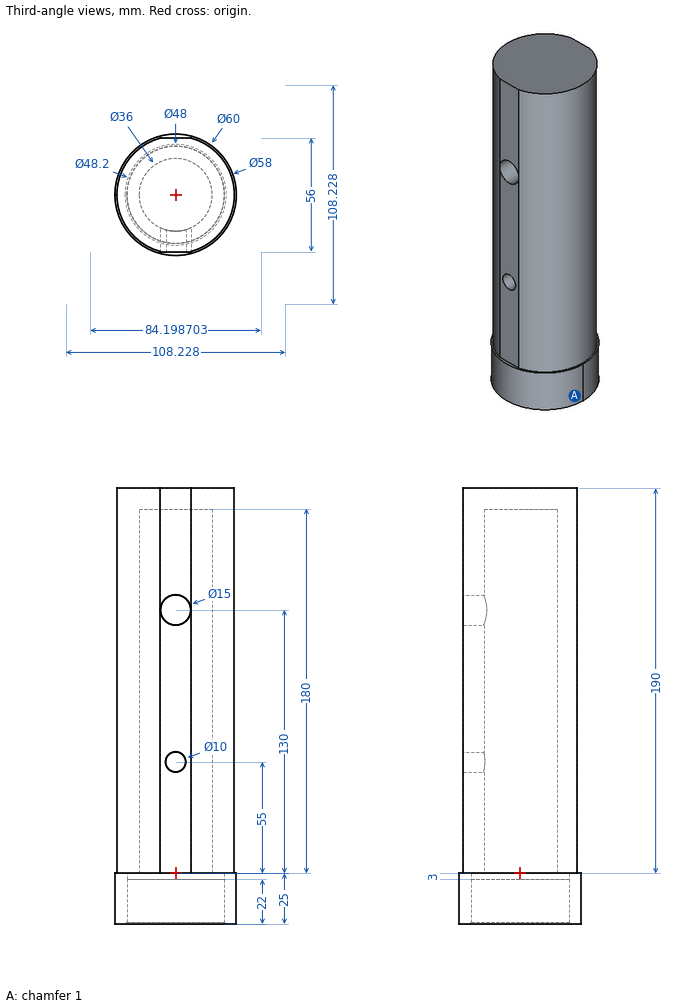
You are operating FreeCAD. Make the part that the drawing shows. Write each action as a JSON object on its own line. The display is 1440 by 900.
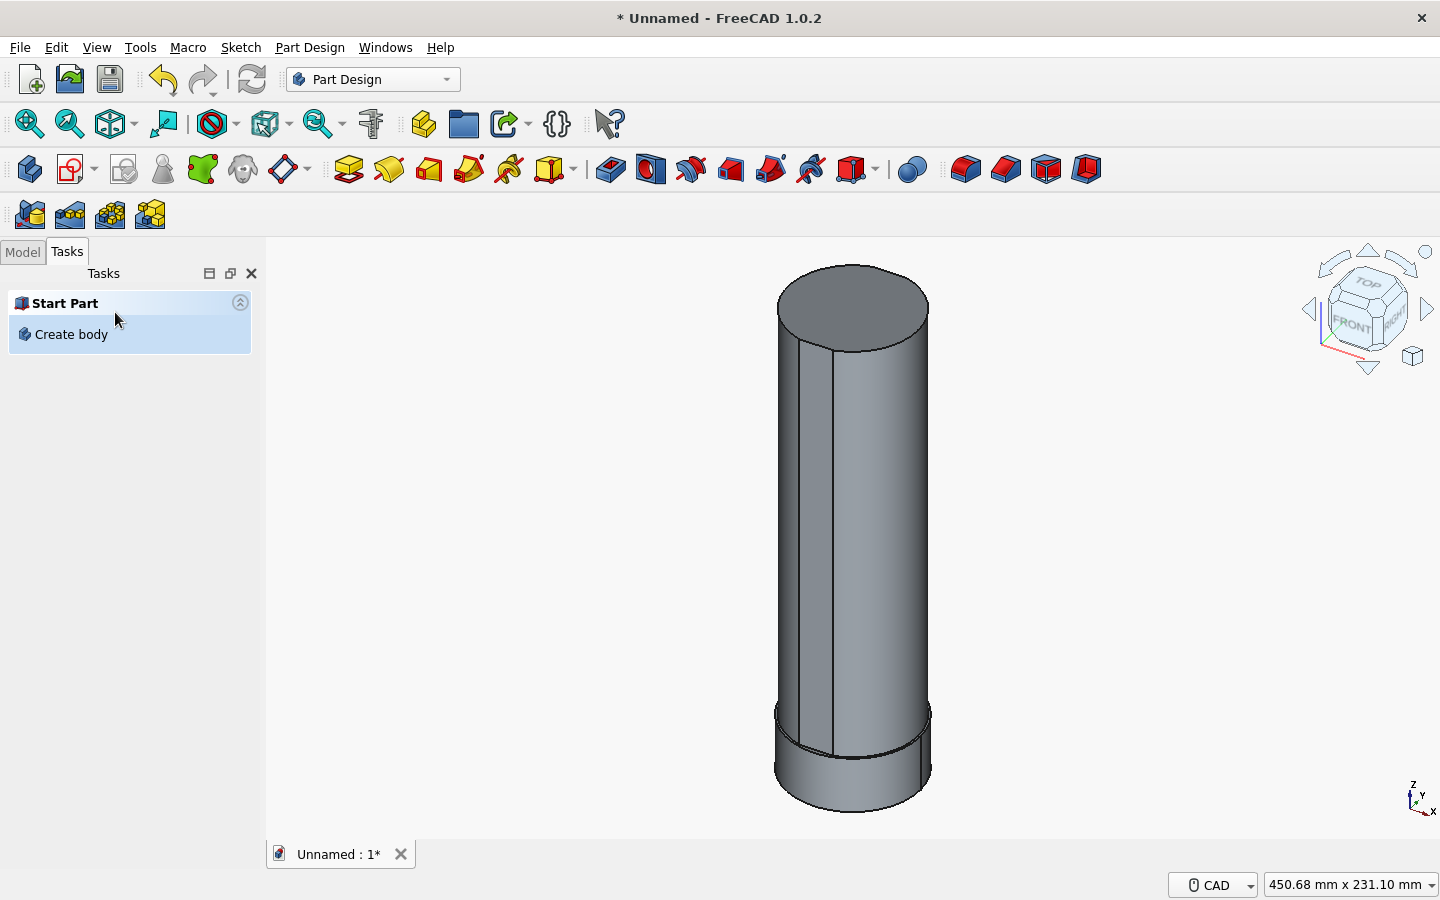
{"action": "key", "text": "5"}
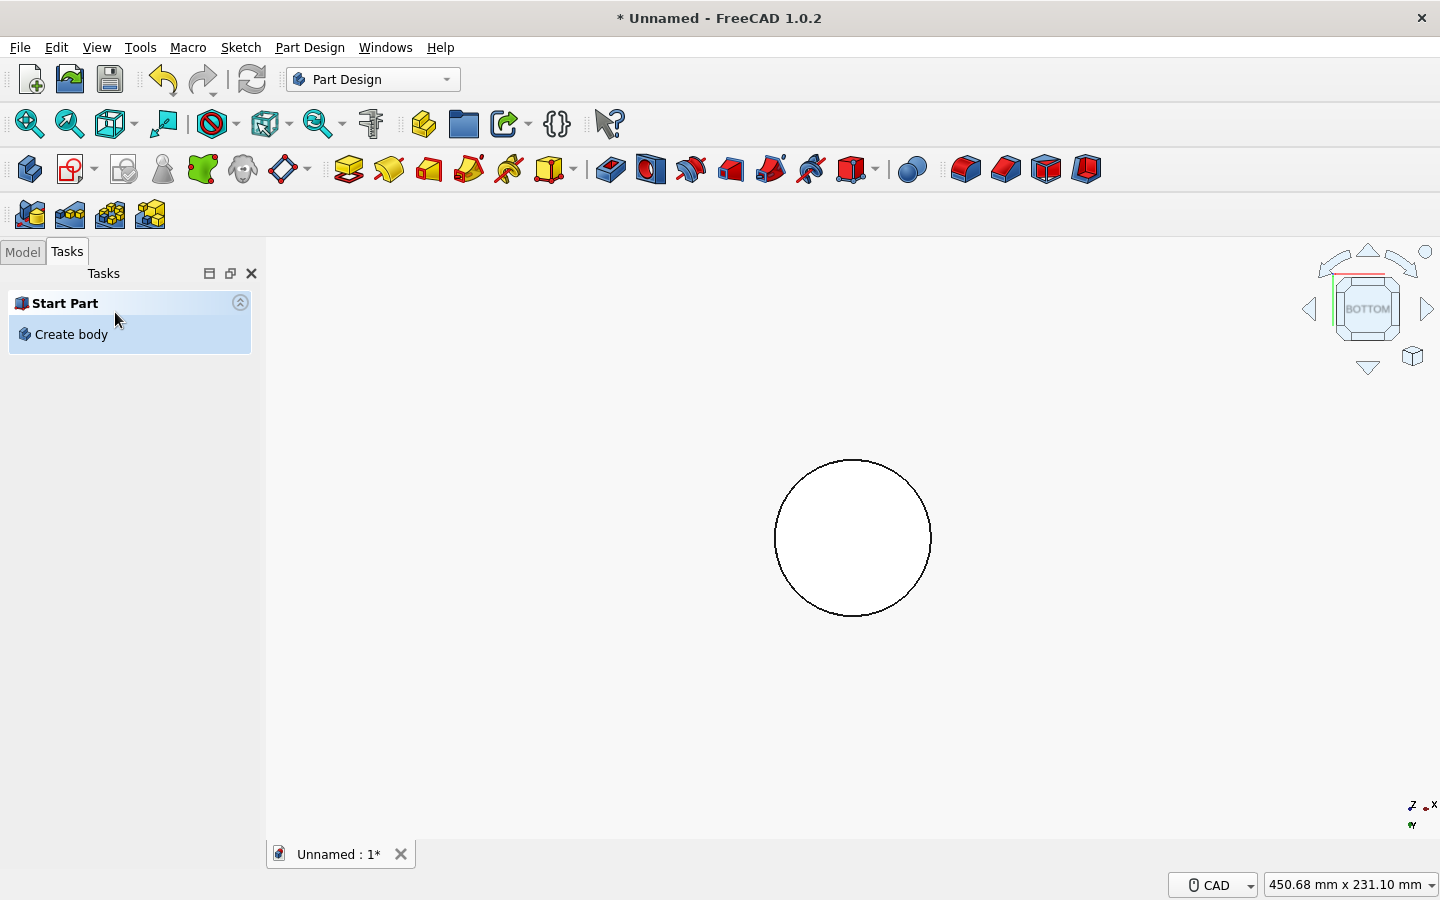
{"action": "left_click", "coordinate": [30, 124]}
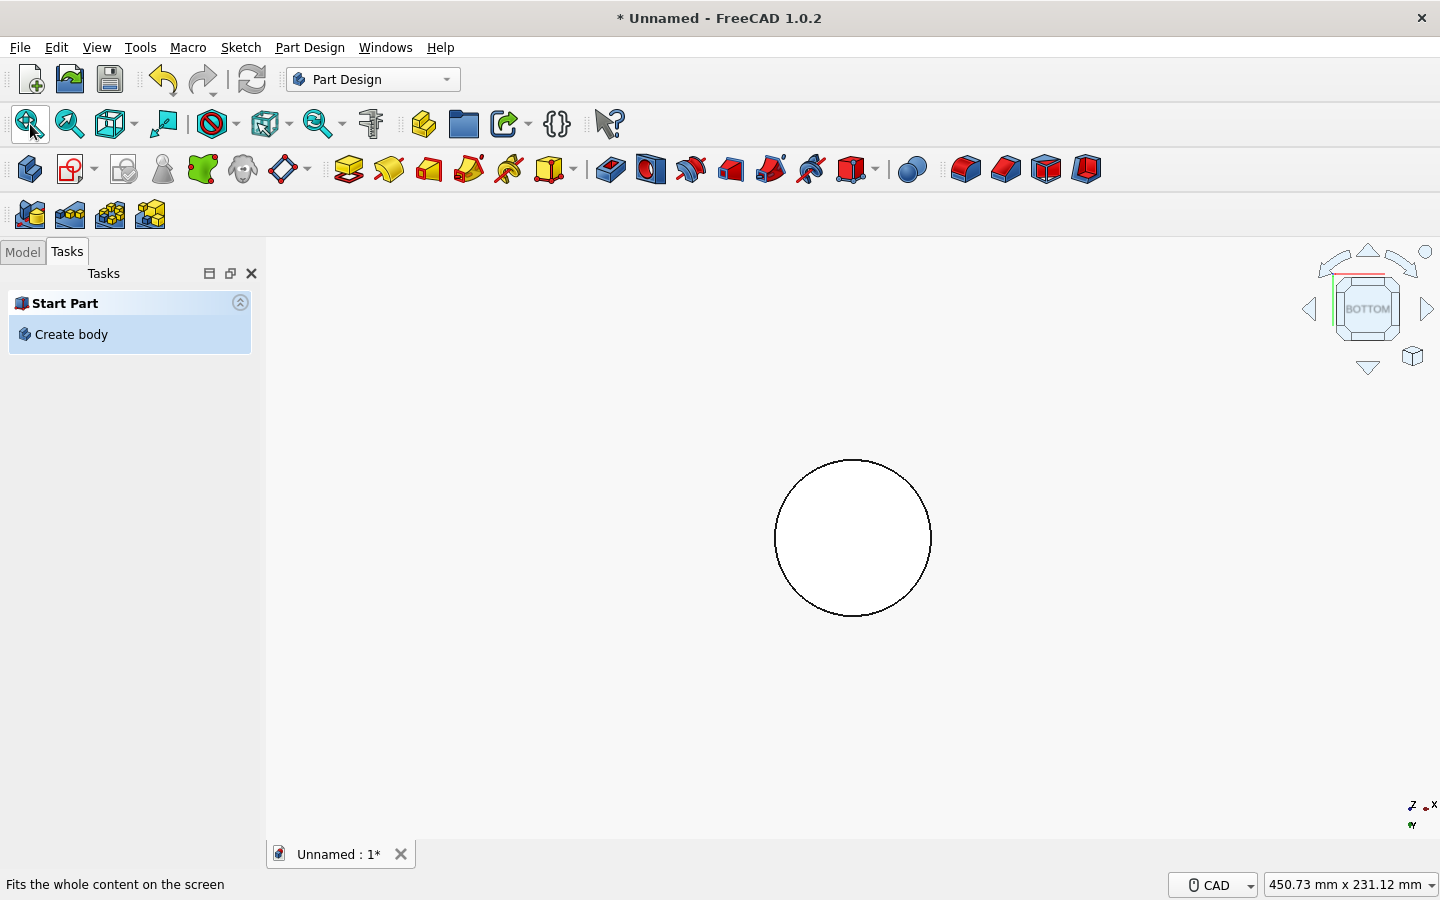
{"action": "left_click", "coordinate": [853, 537]}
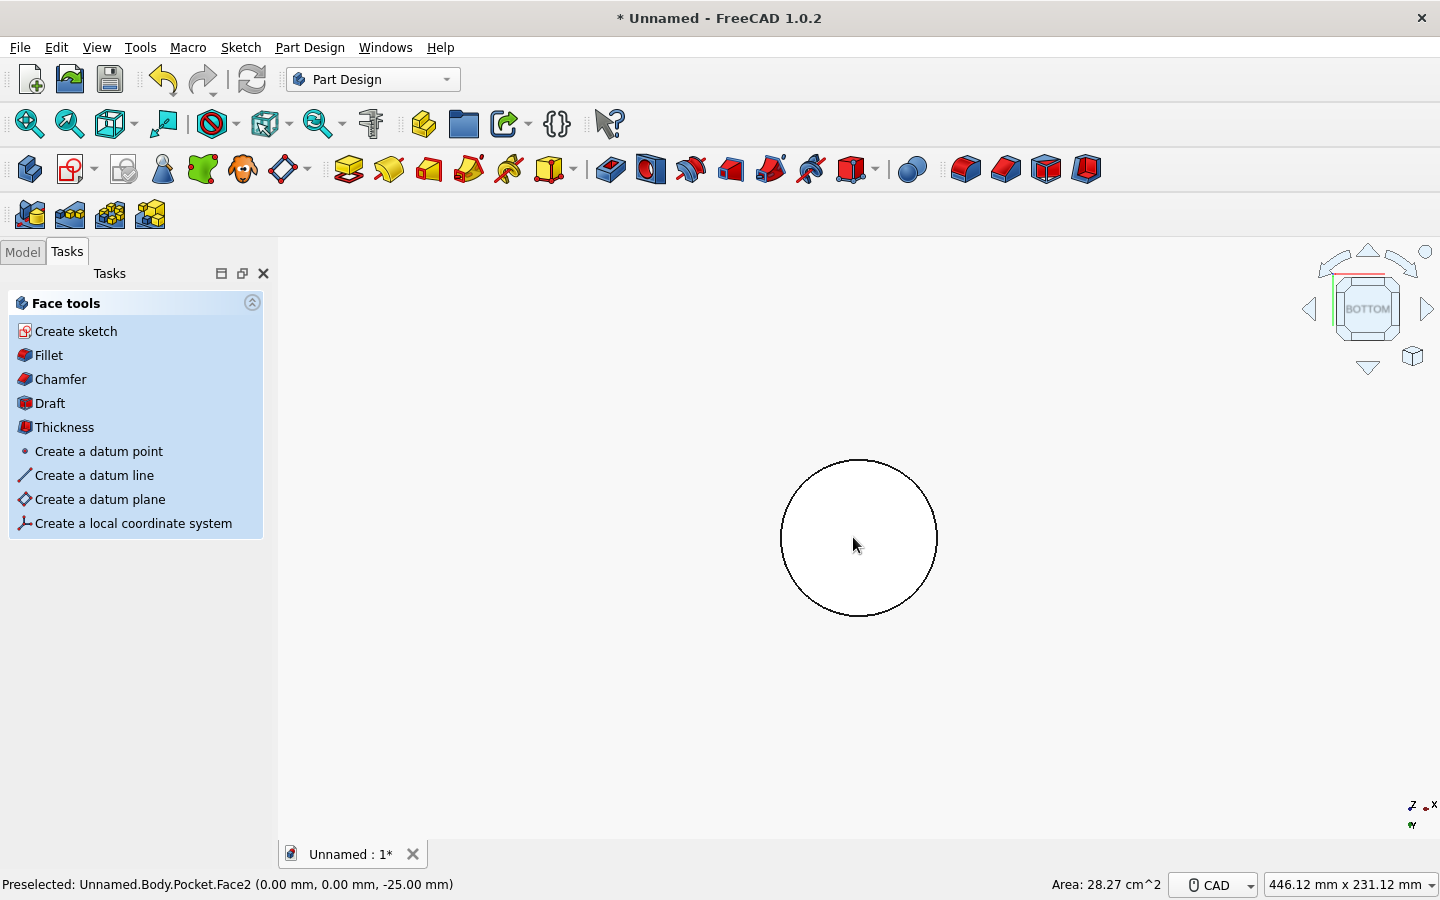
{"action": "left_click", "coordinate": [70, 170]}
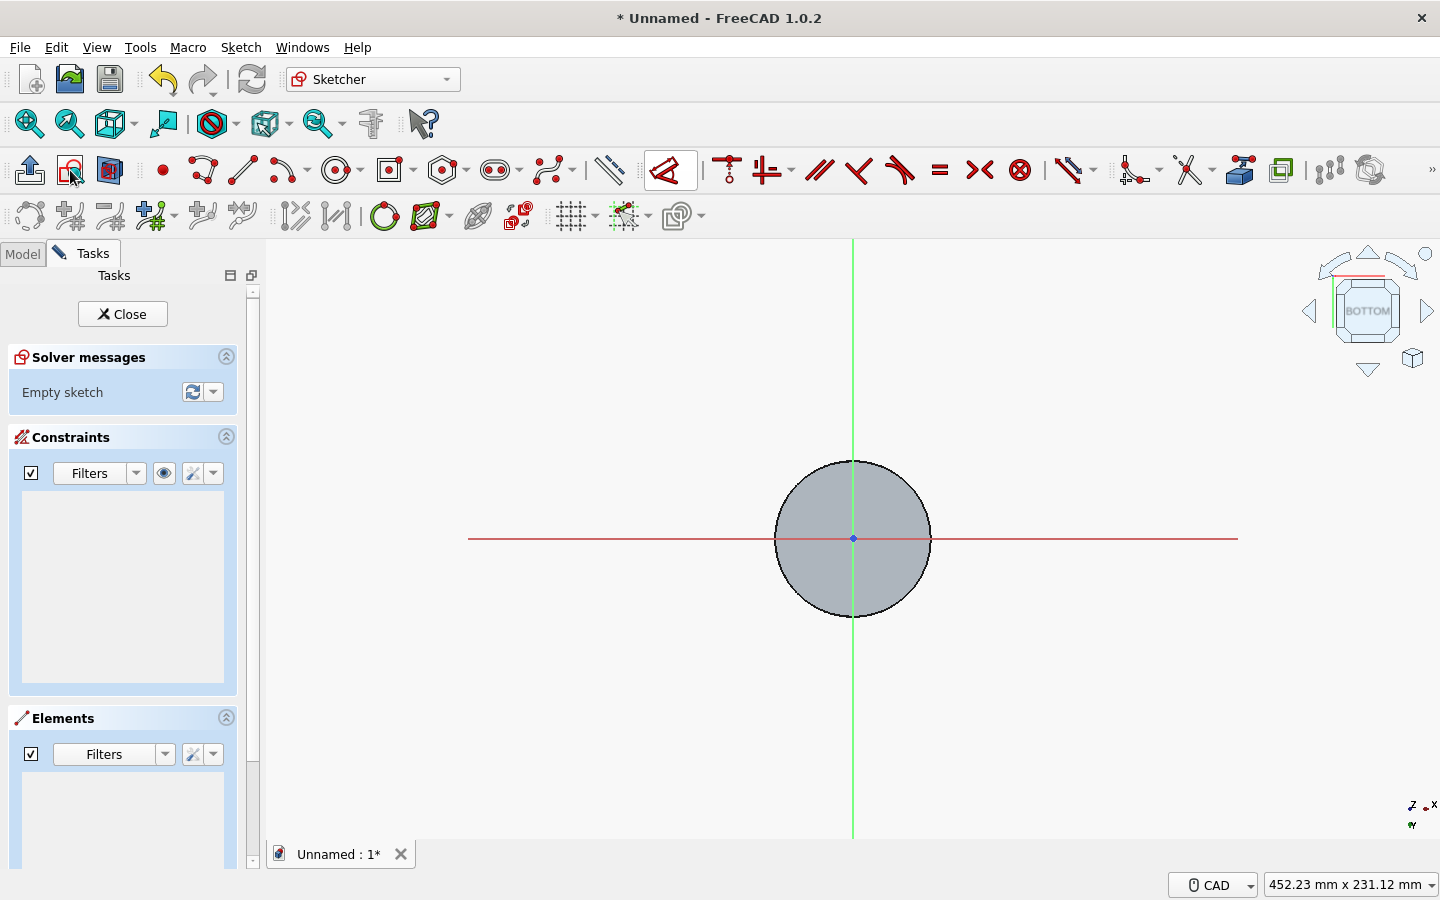
{"action": "scroll", "coordinate": [883, 539], "scroll_direction": "up", "scroll_amount": 6}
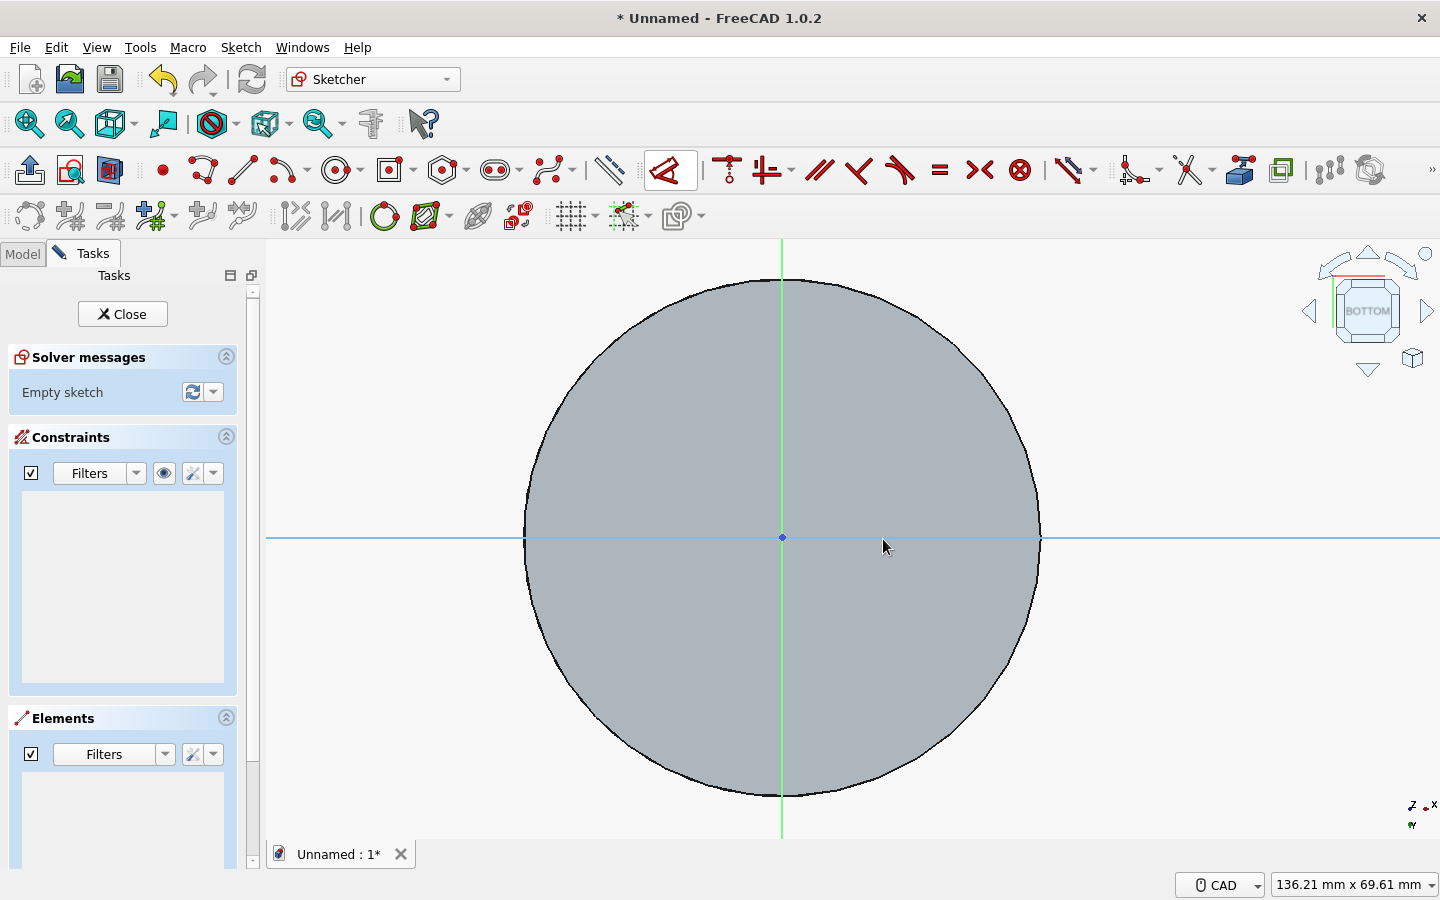
{"action": "left_click", "coordinate": [336, 170]}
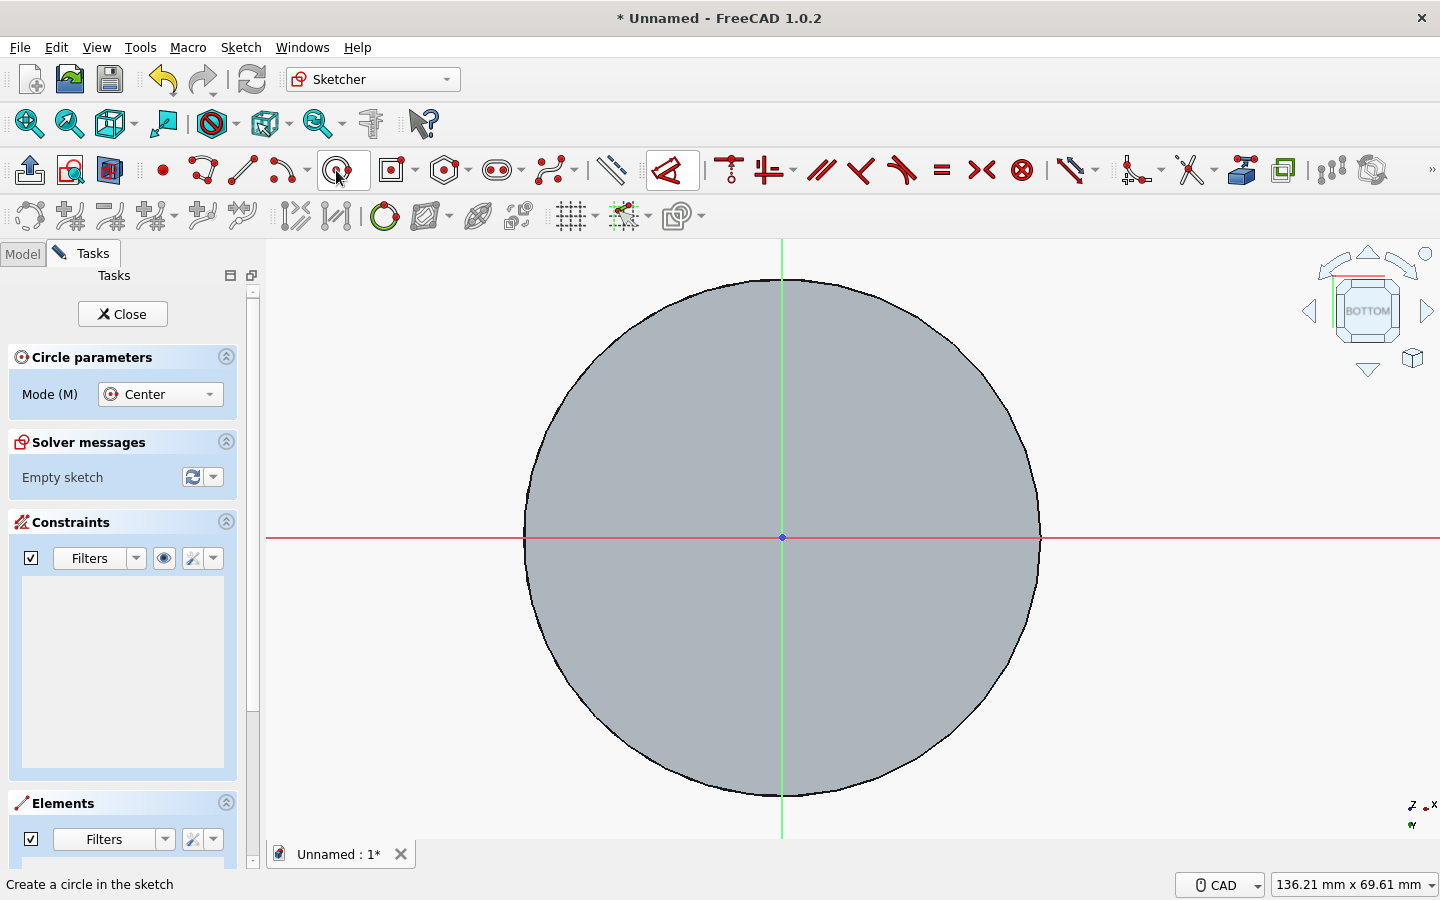
{"action": "left_click", "coordinate": [782, 538]}
{"action": "left_click", "coordinate": [928, 392]}
{"action": "key", "text": "Escape"}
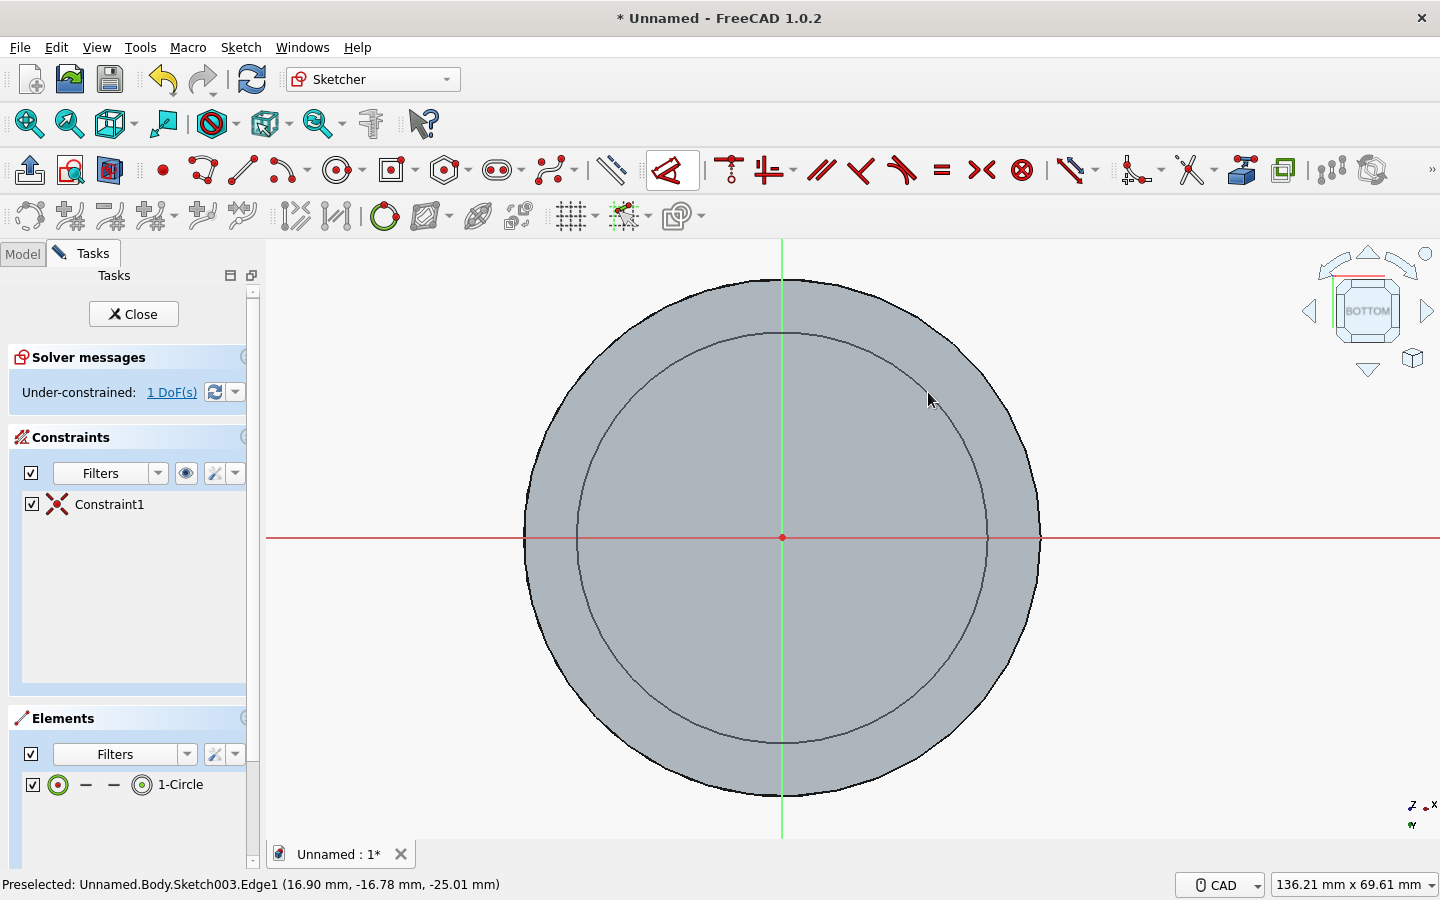
{"action": "left_click", "coordinate": [927, 392]}